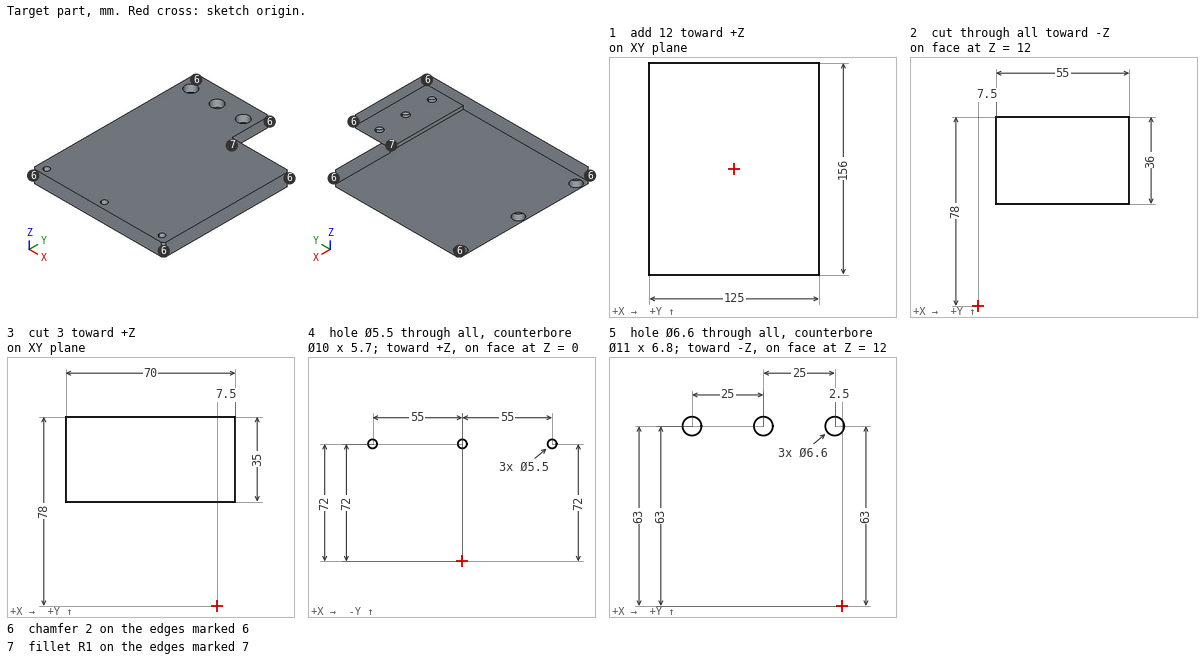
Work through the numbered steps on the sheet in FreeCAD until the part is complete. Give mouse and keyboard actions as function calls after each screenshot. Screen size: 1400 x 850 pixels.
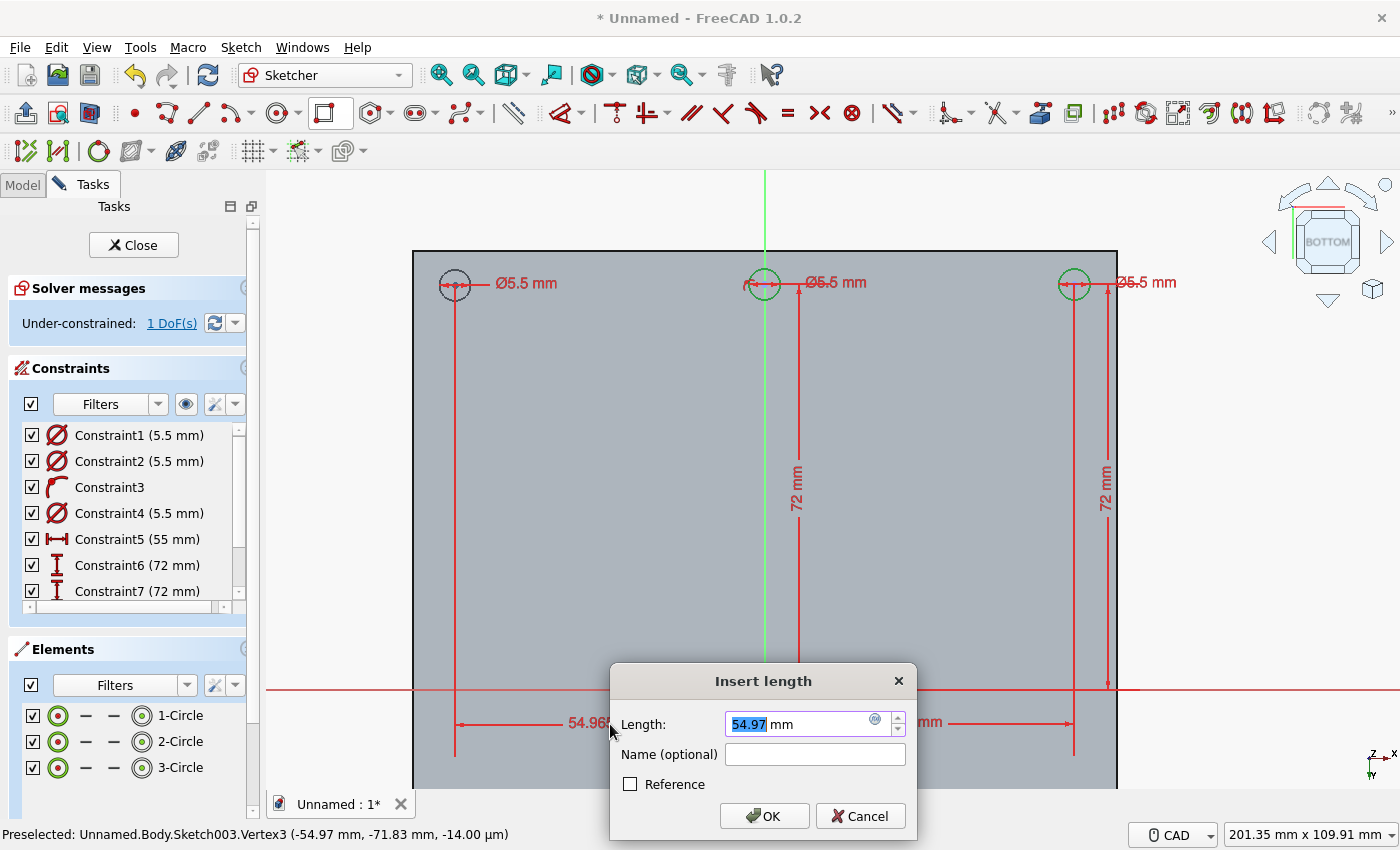
text(55)
key(Return)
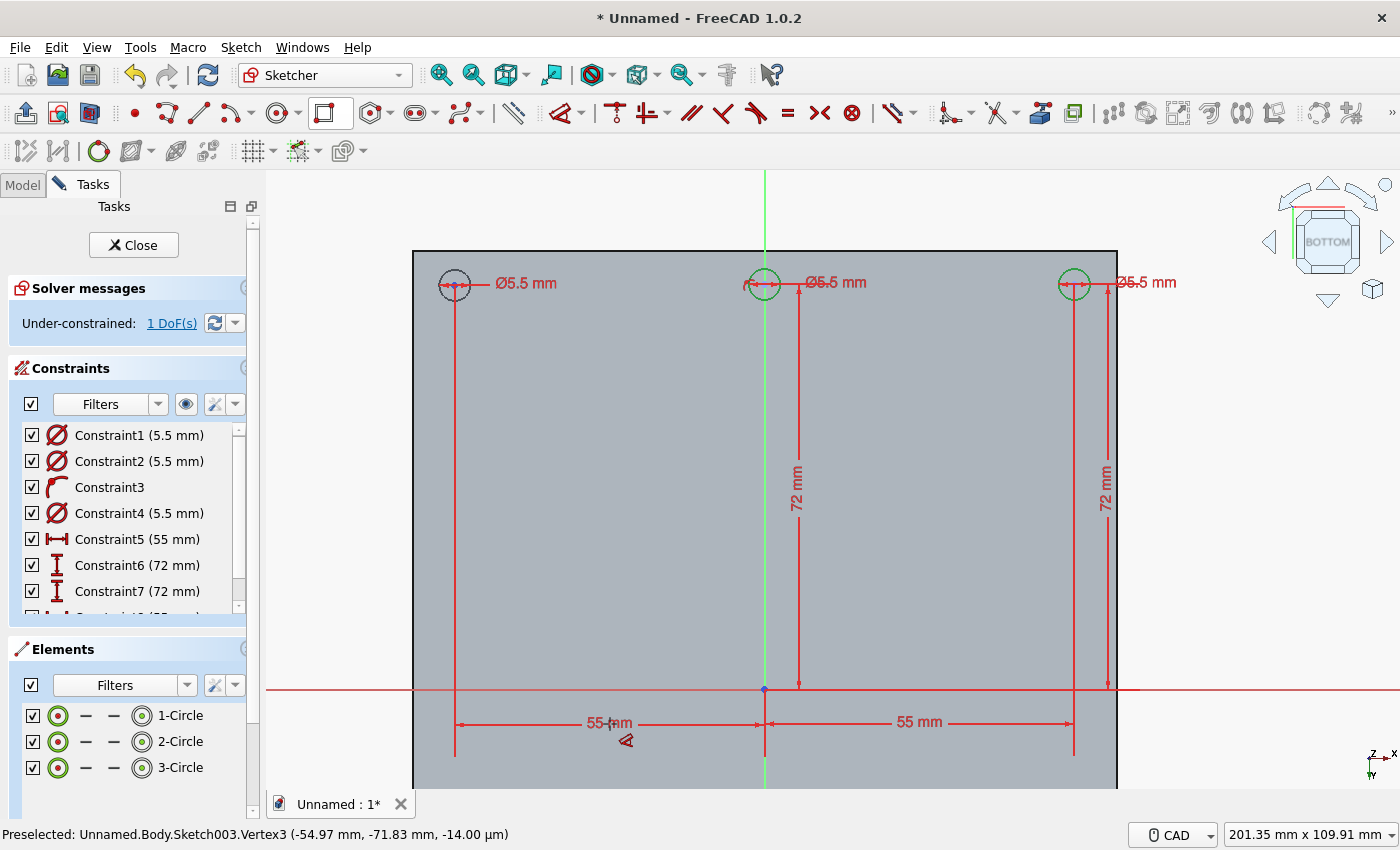
click(455, 285)
click(421, 488)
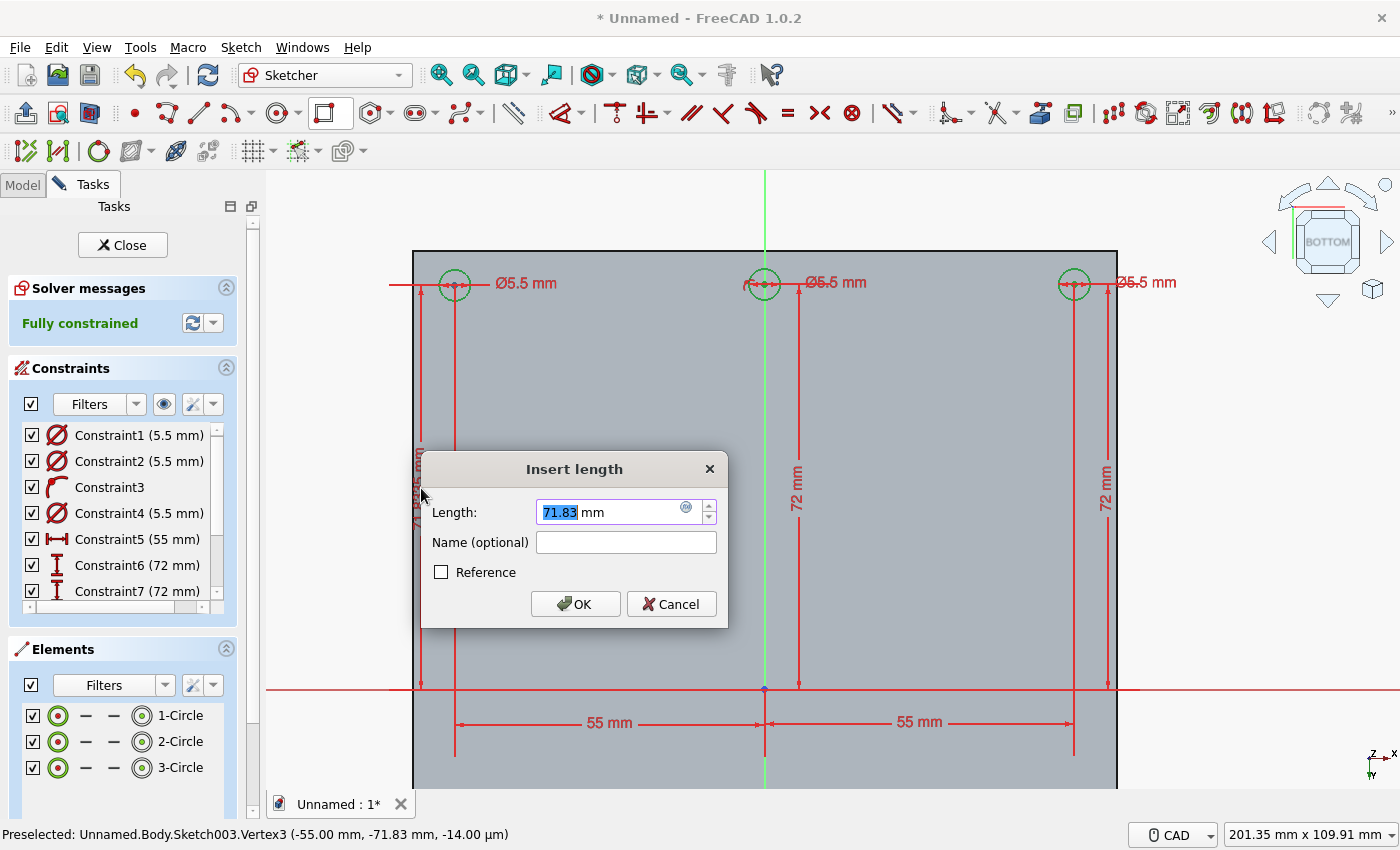
text(72)
key(Return)
key(Escape)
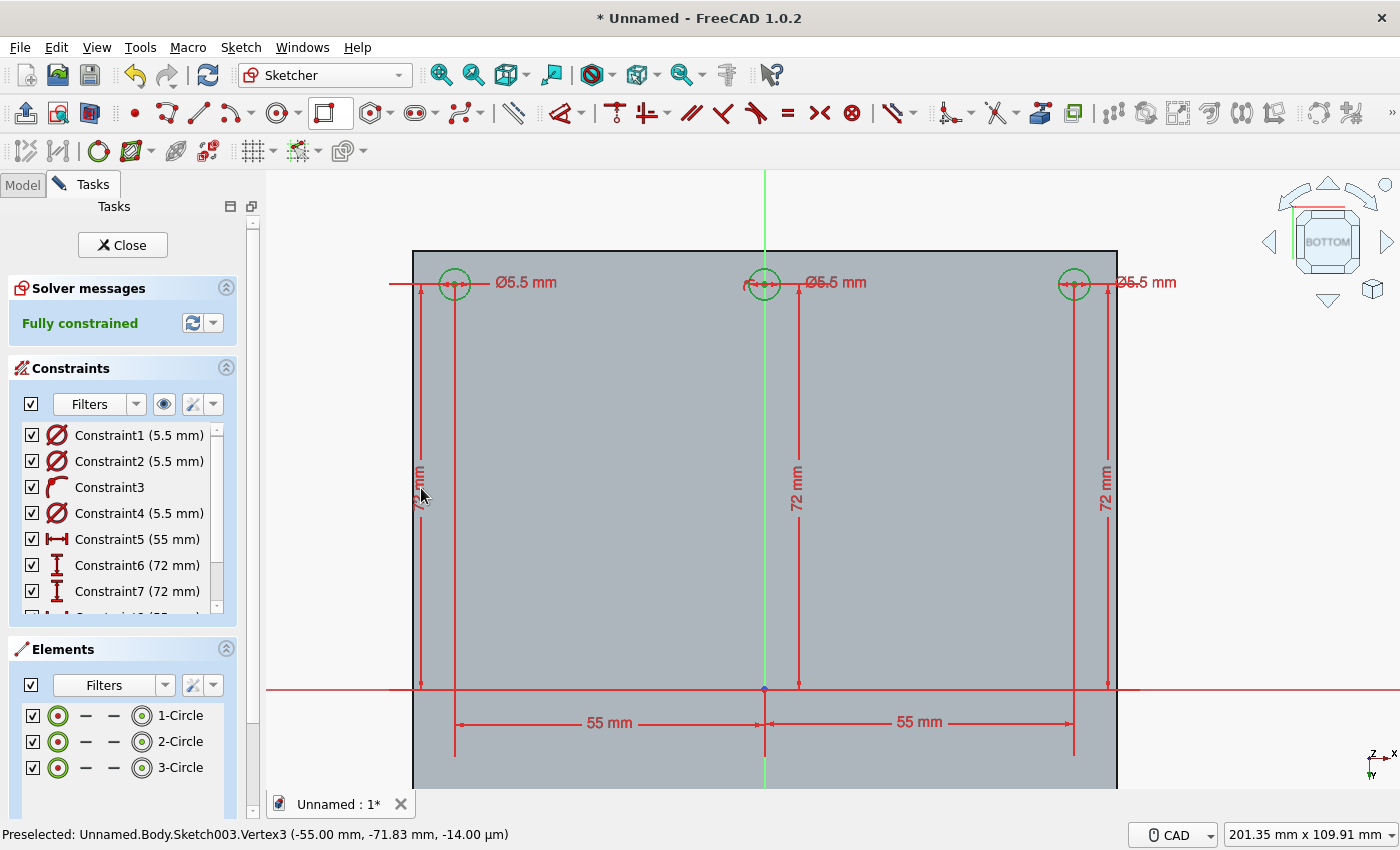
click(123, 245)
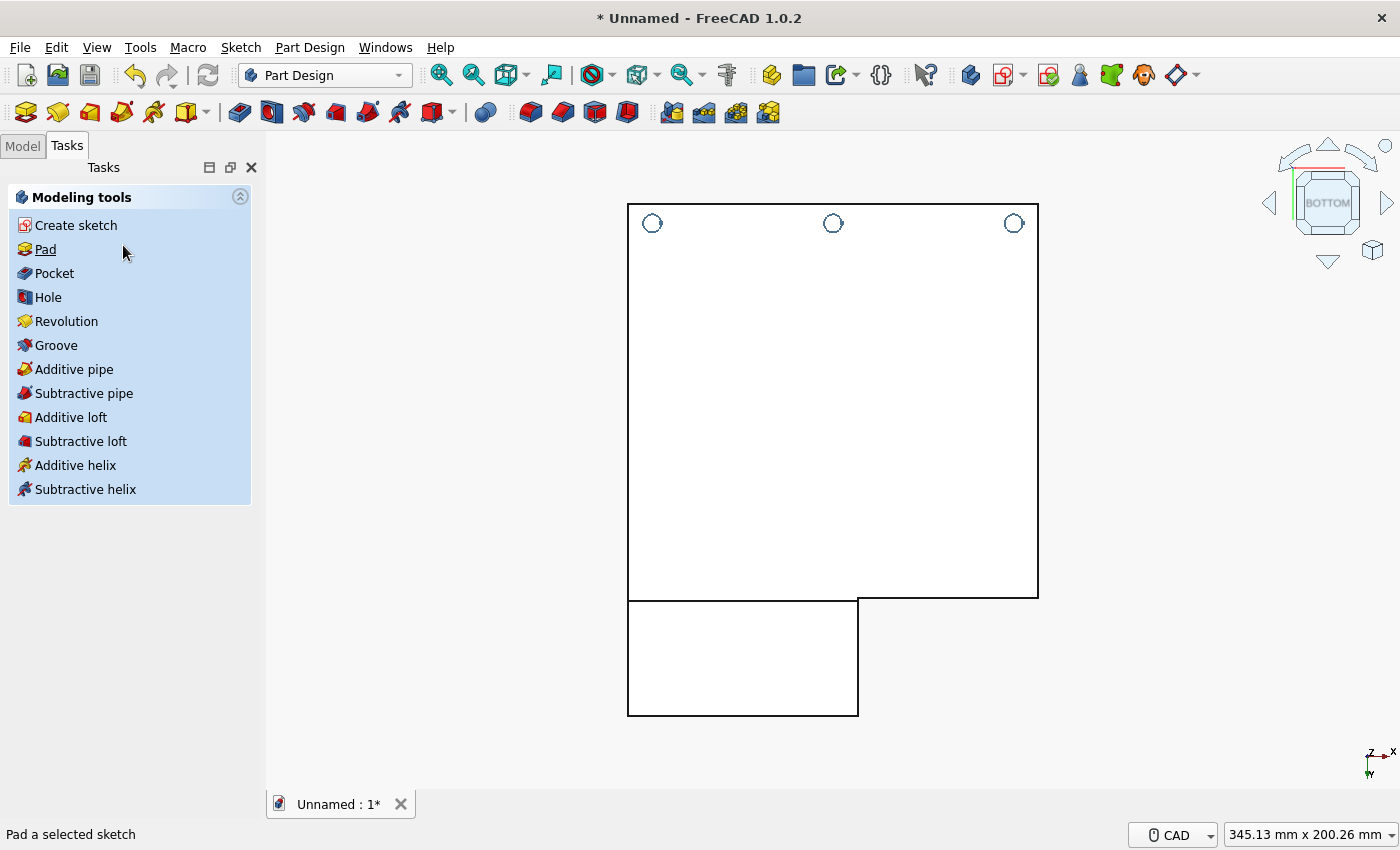
click(272, 112)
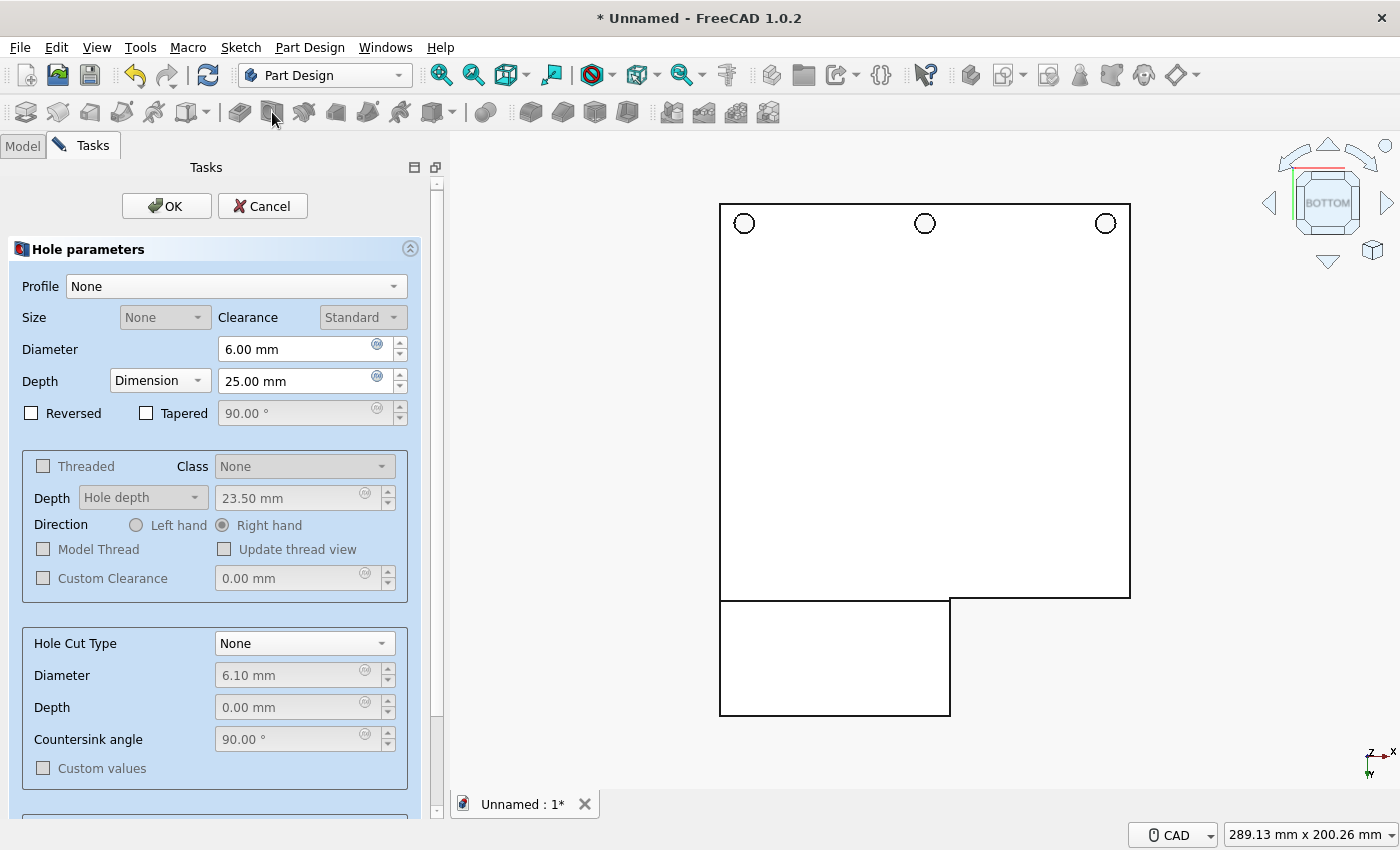
triple_click(305, 349)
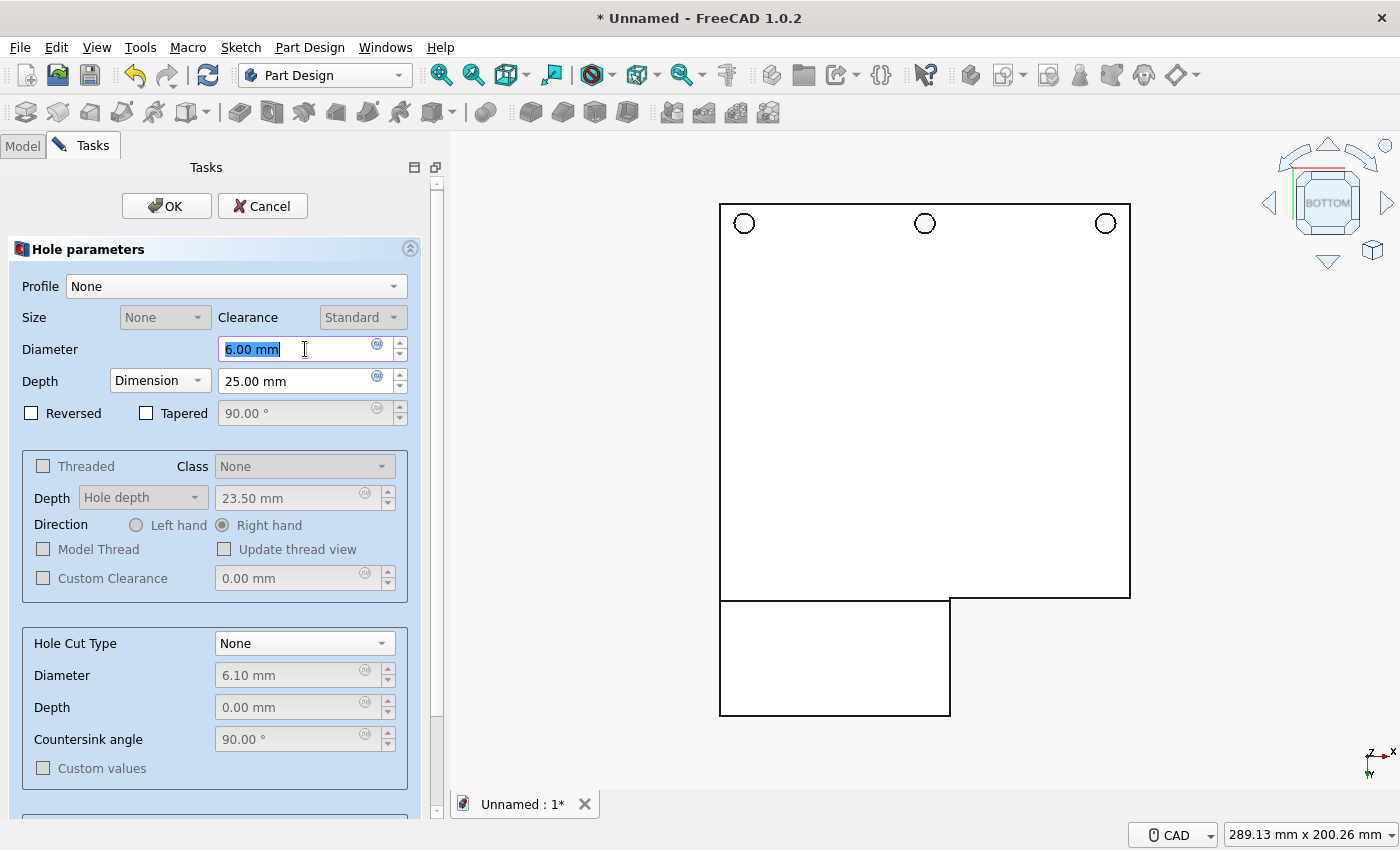
text(5.5)
key(Tab)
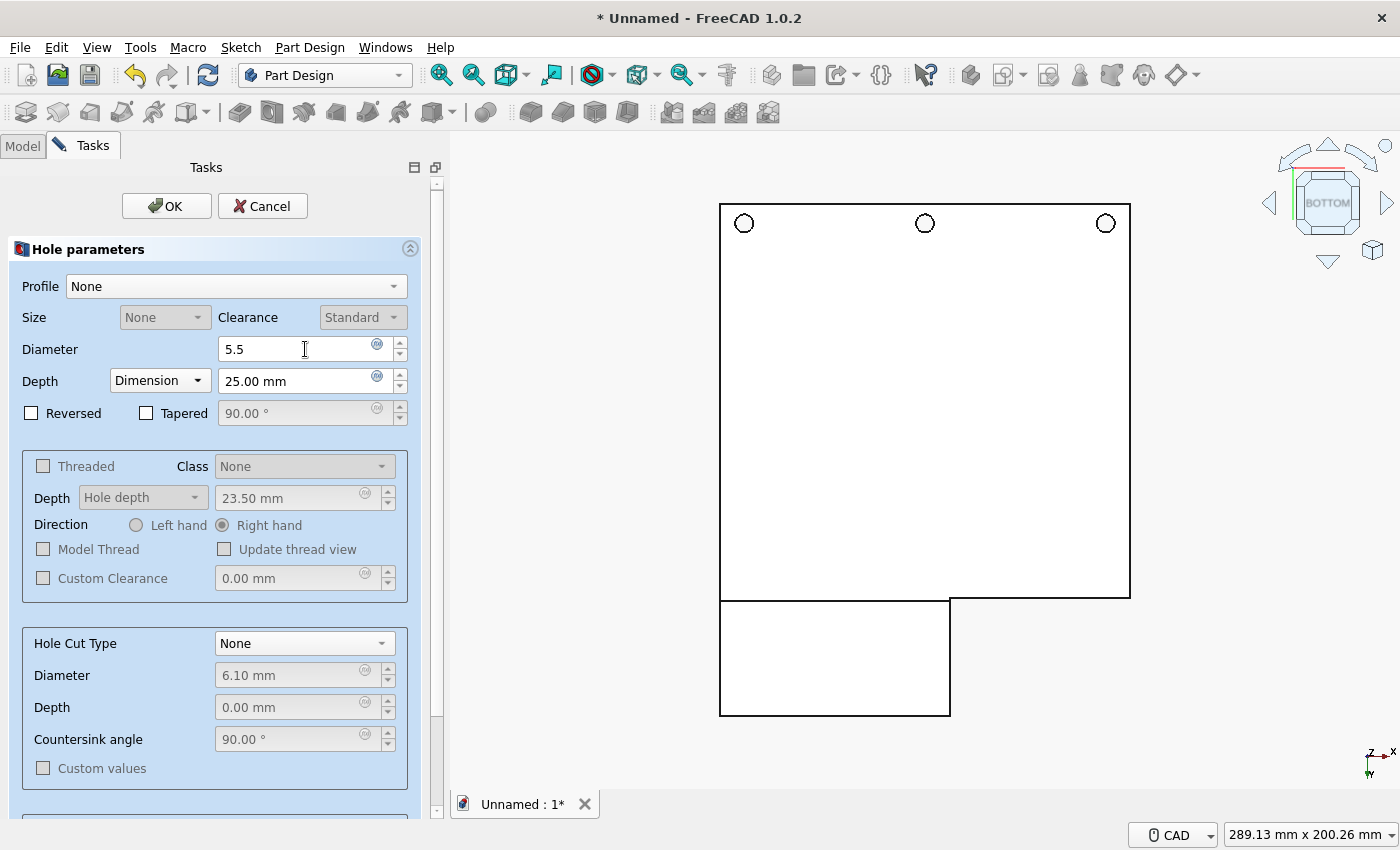
click(161, 380)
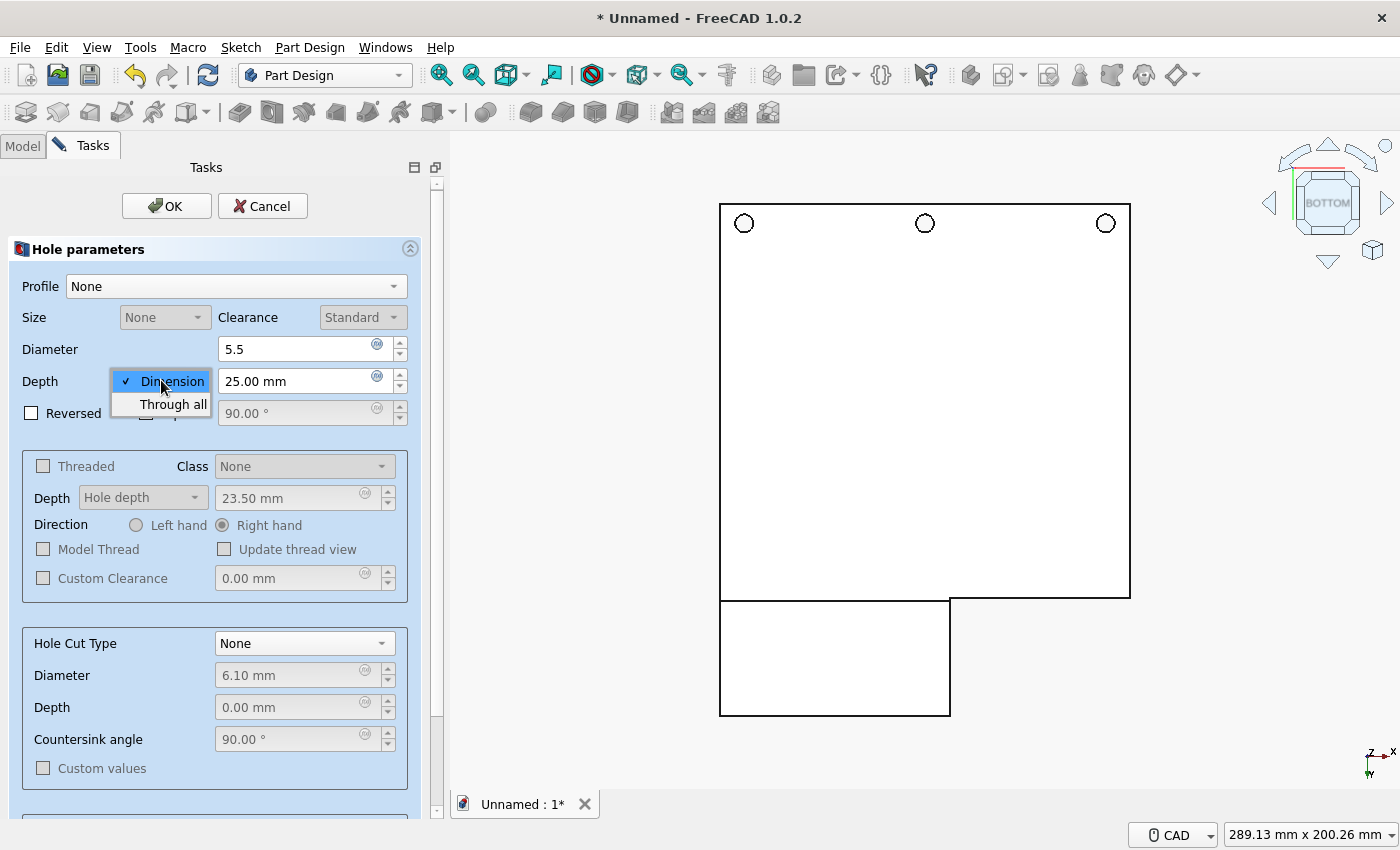
click(160, 404)